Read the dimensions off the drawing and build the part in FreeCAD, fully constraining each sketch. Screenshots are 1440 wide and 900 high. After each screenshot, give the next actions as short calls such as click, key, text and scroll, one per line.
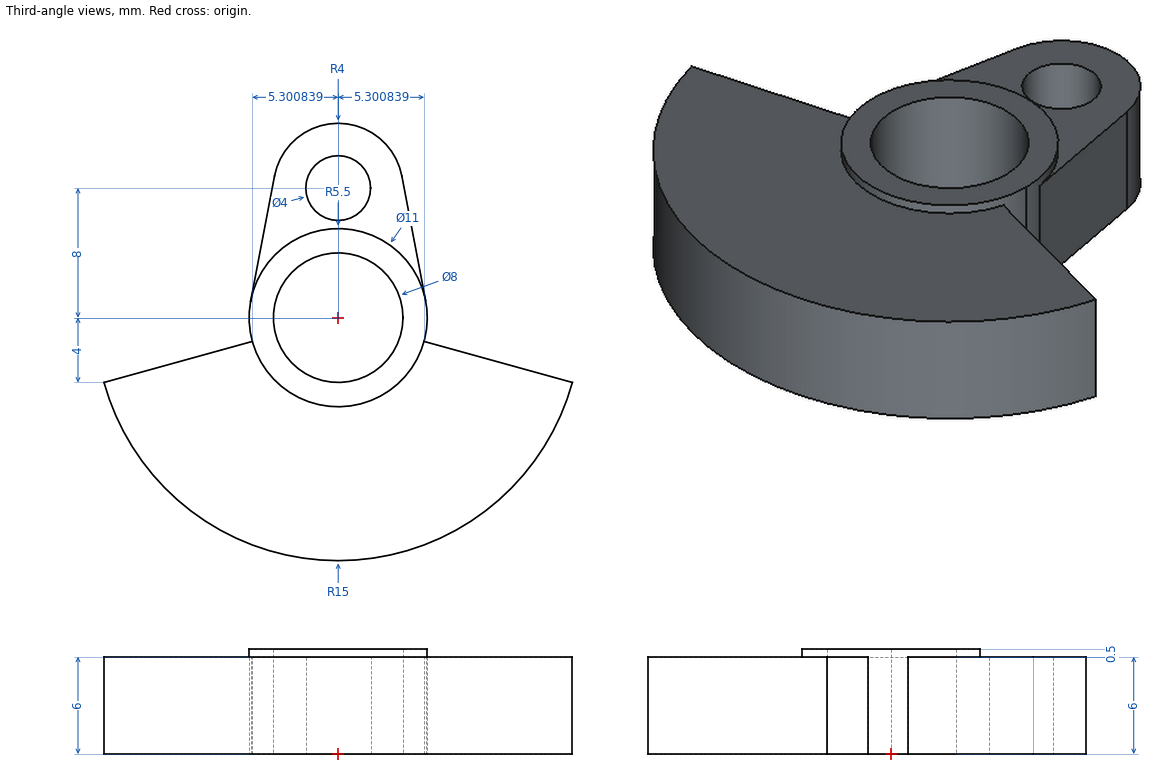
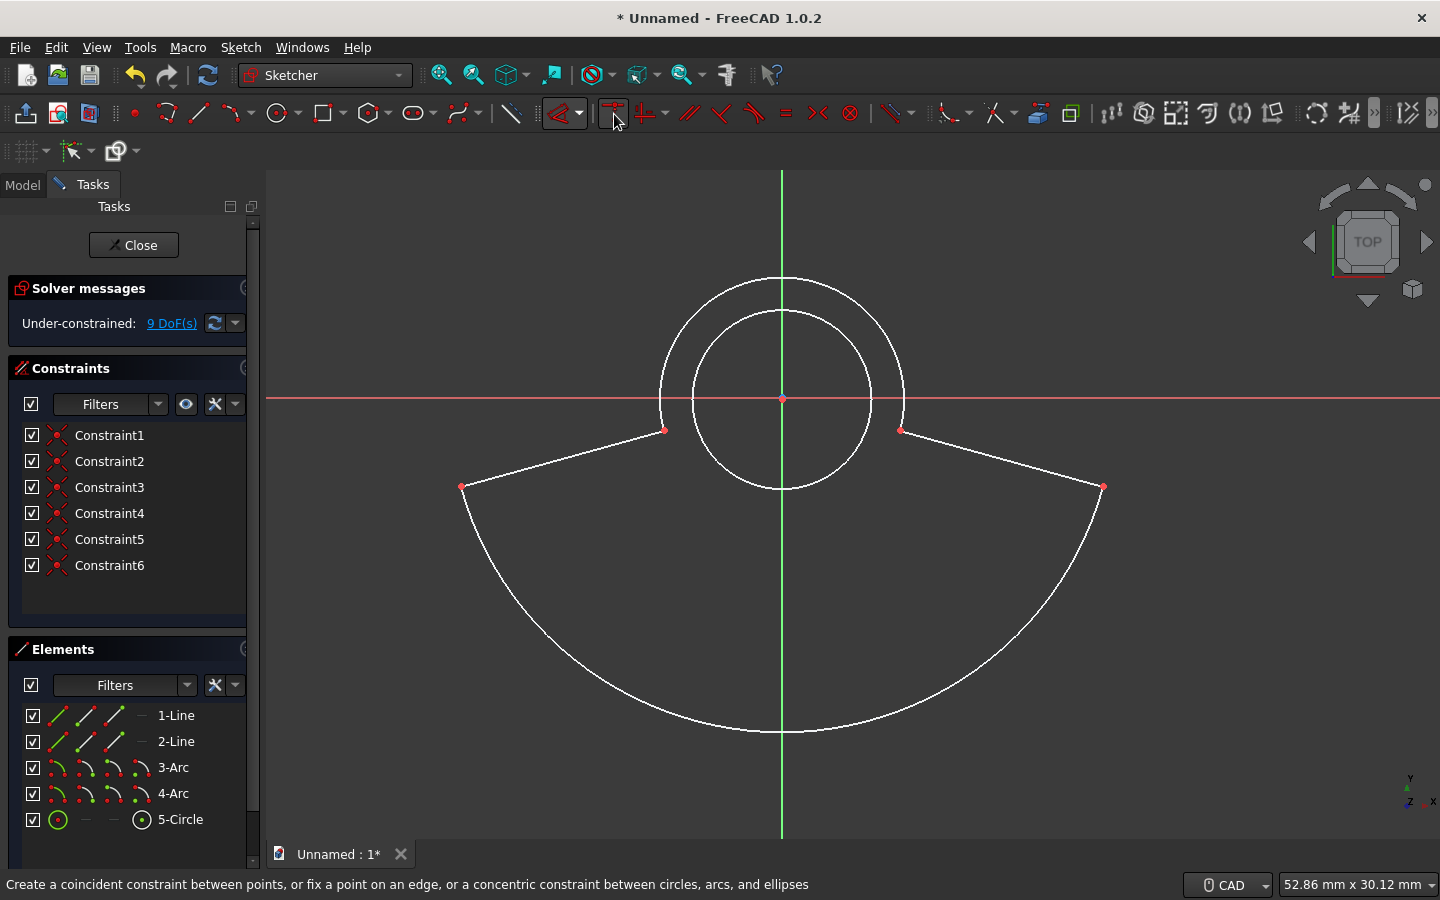
drag(772, 388, 792, 410)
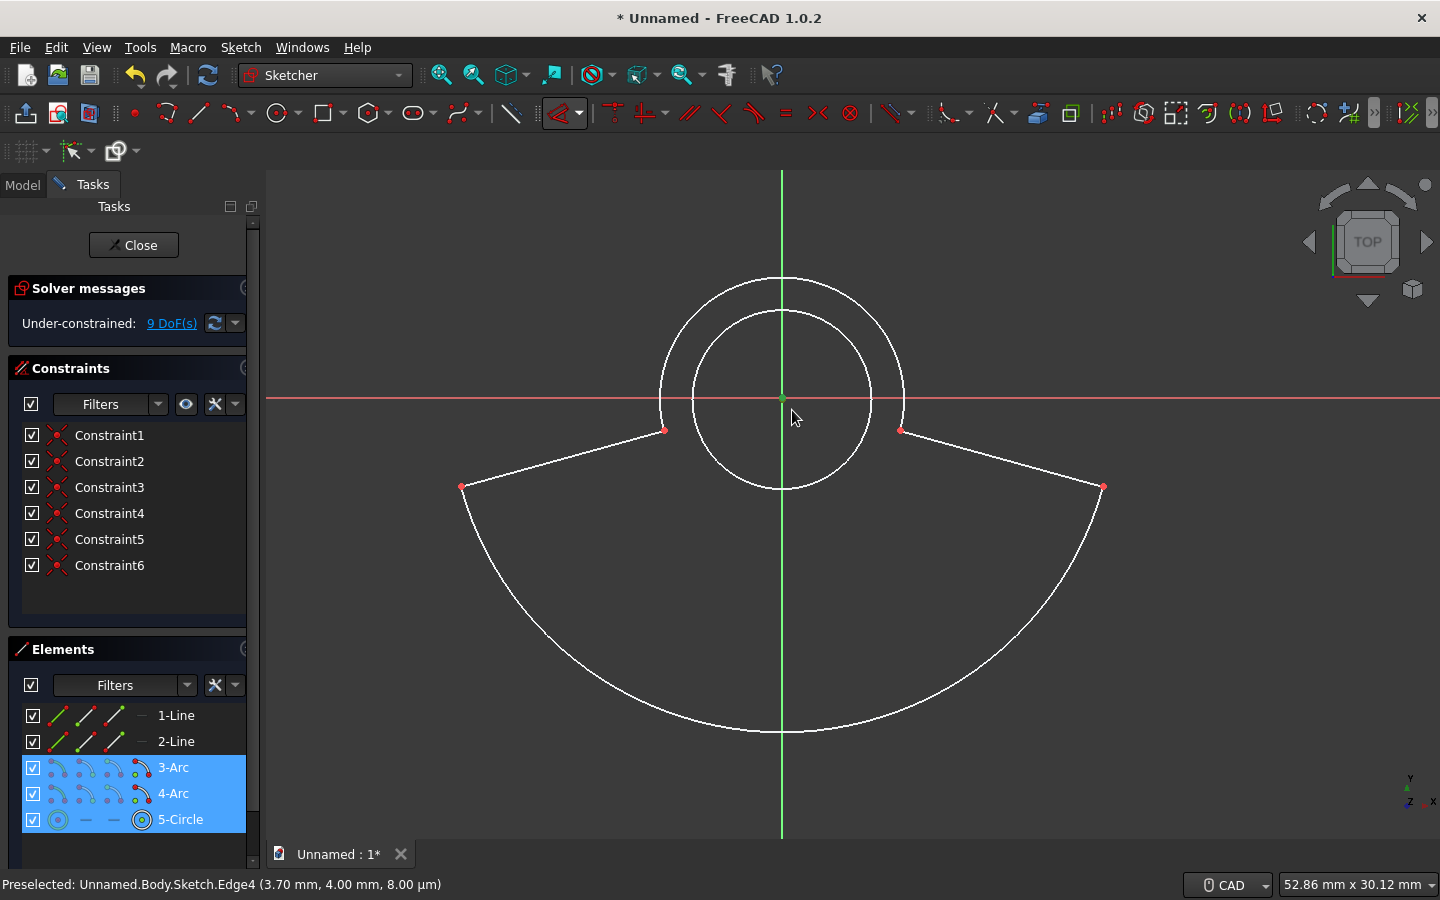
click(614, 114)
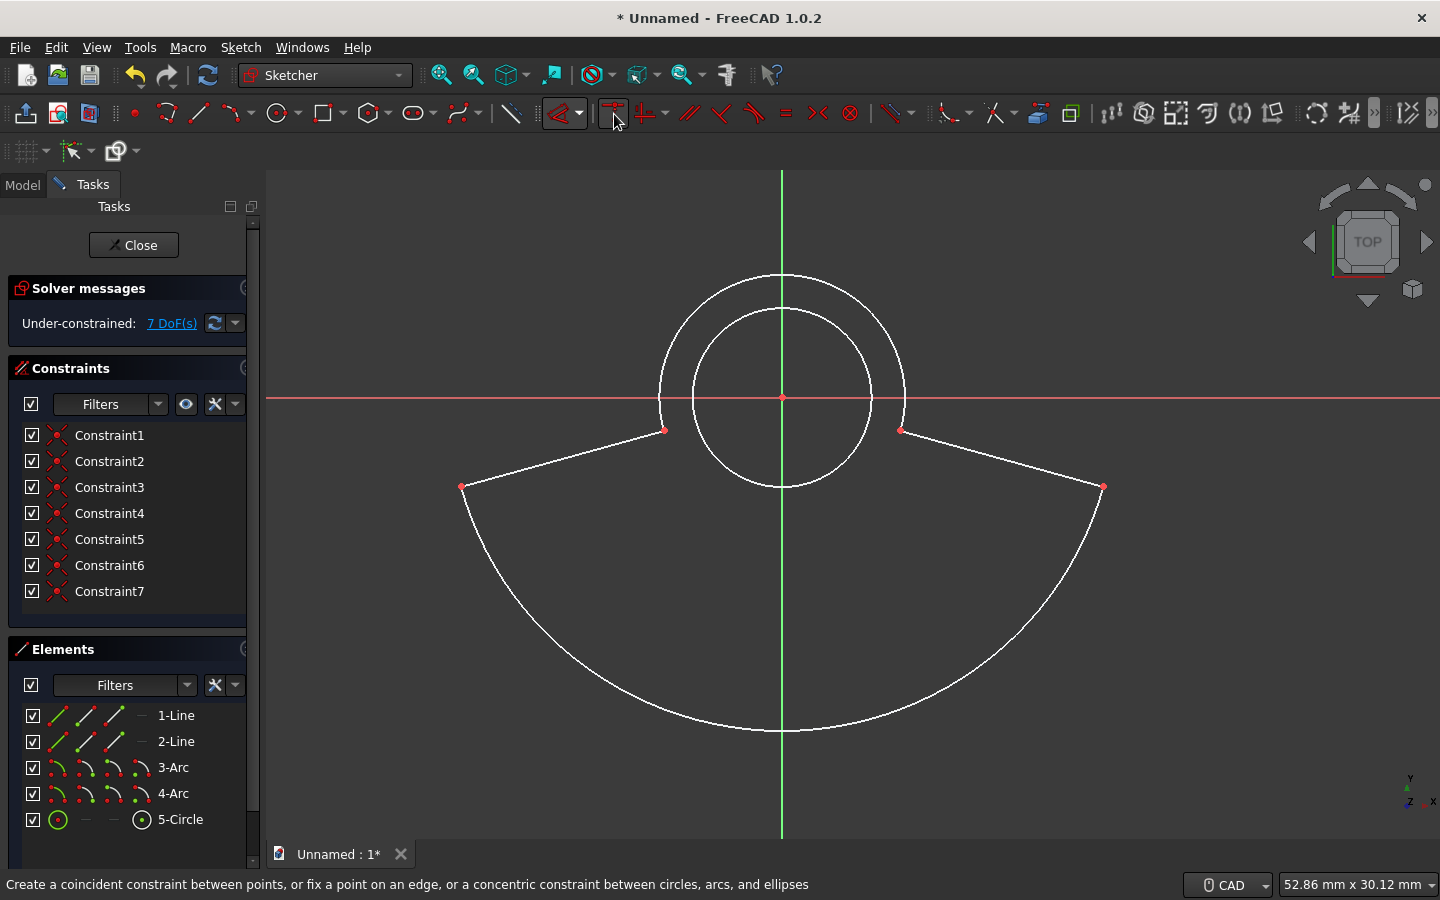
click(558, 114)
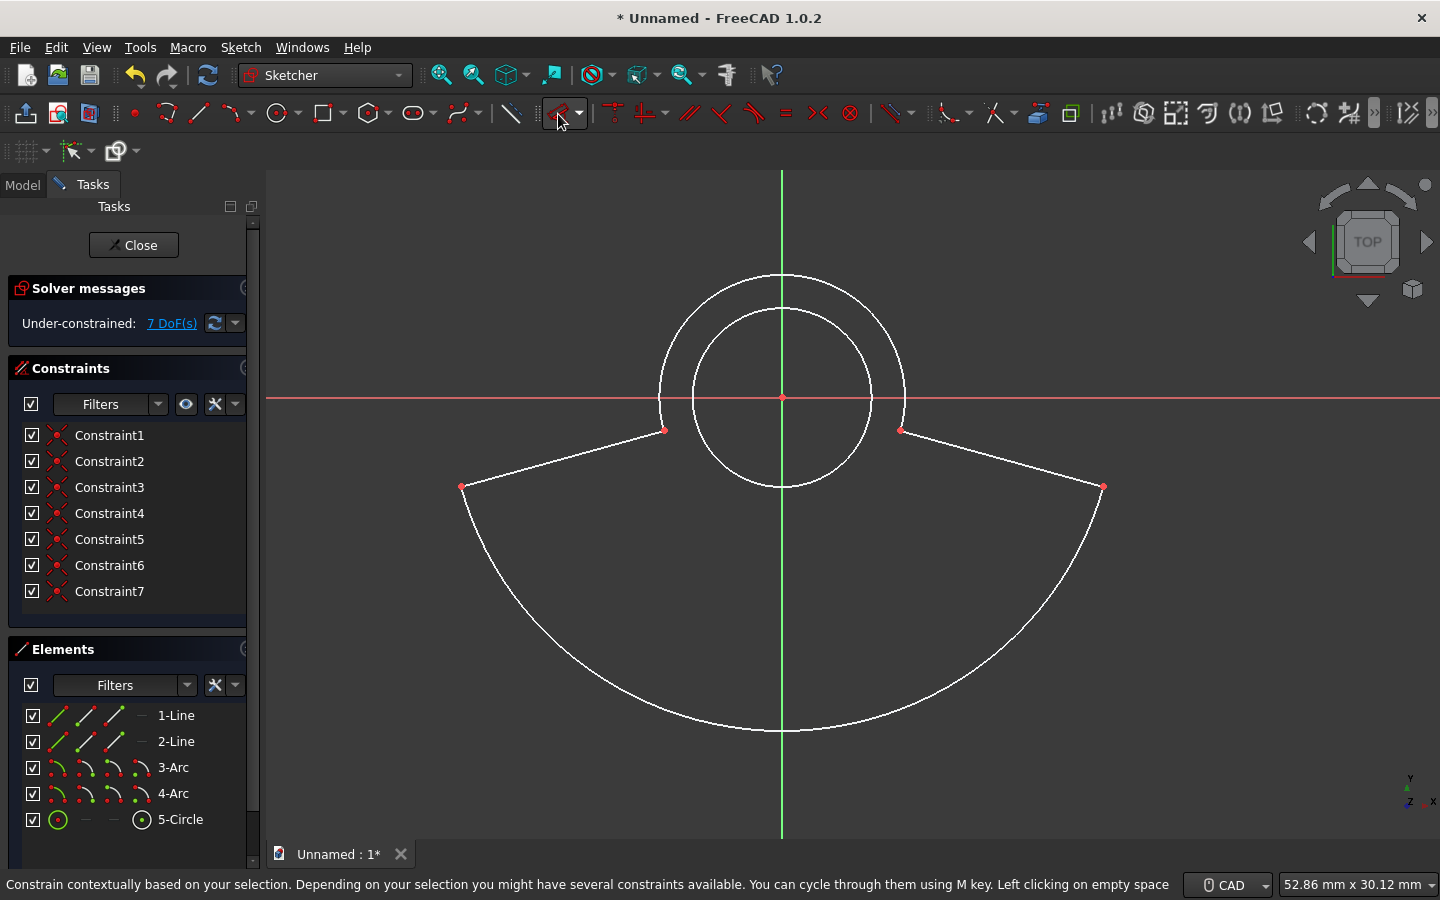
click(617, 687)
click(601, 715)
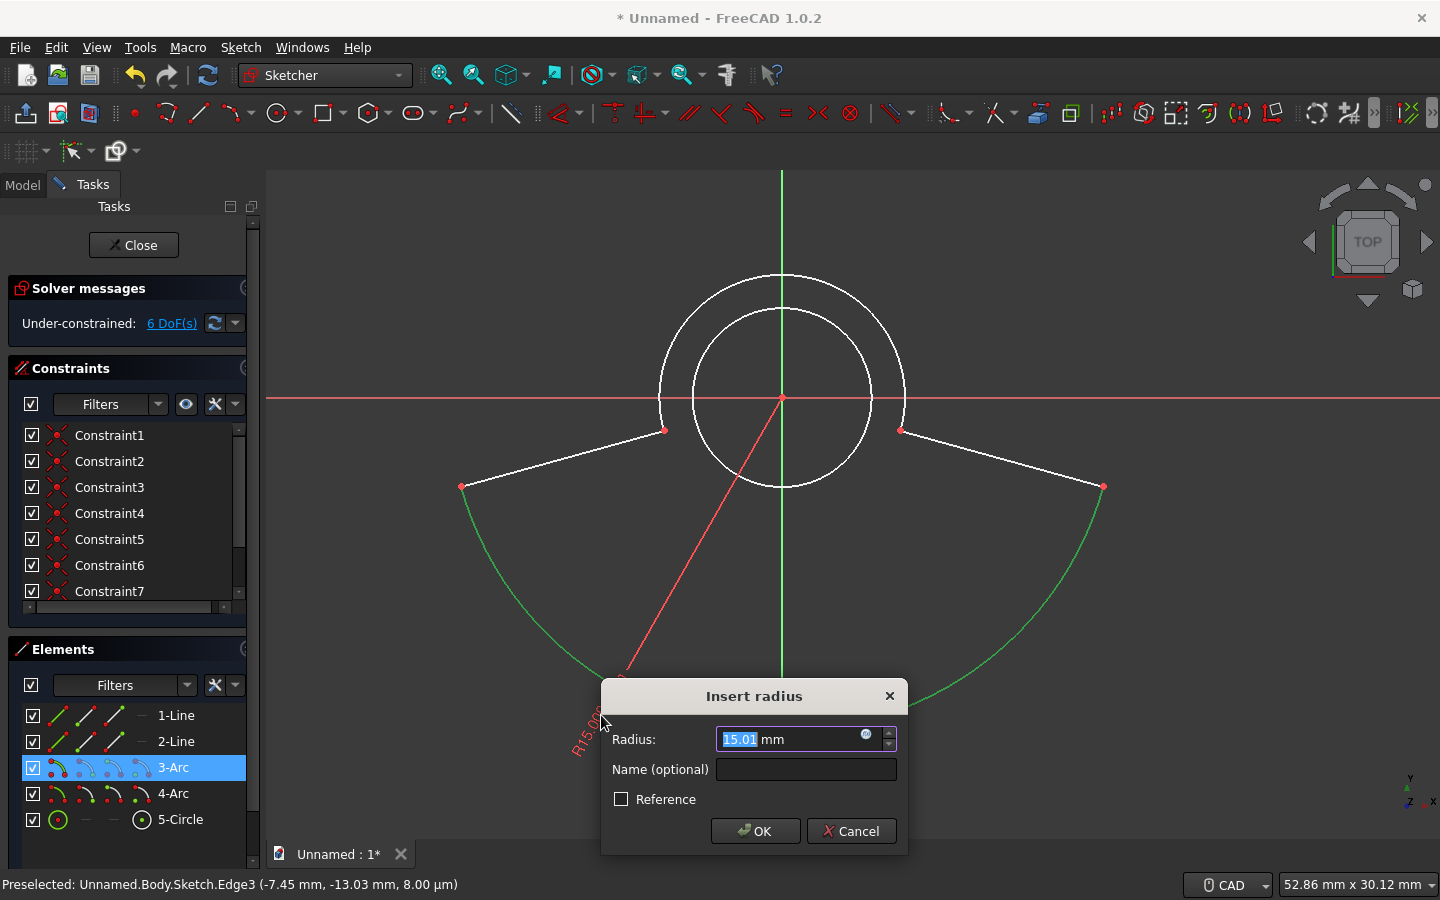
text(15)
key(Return)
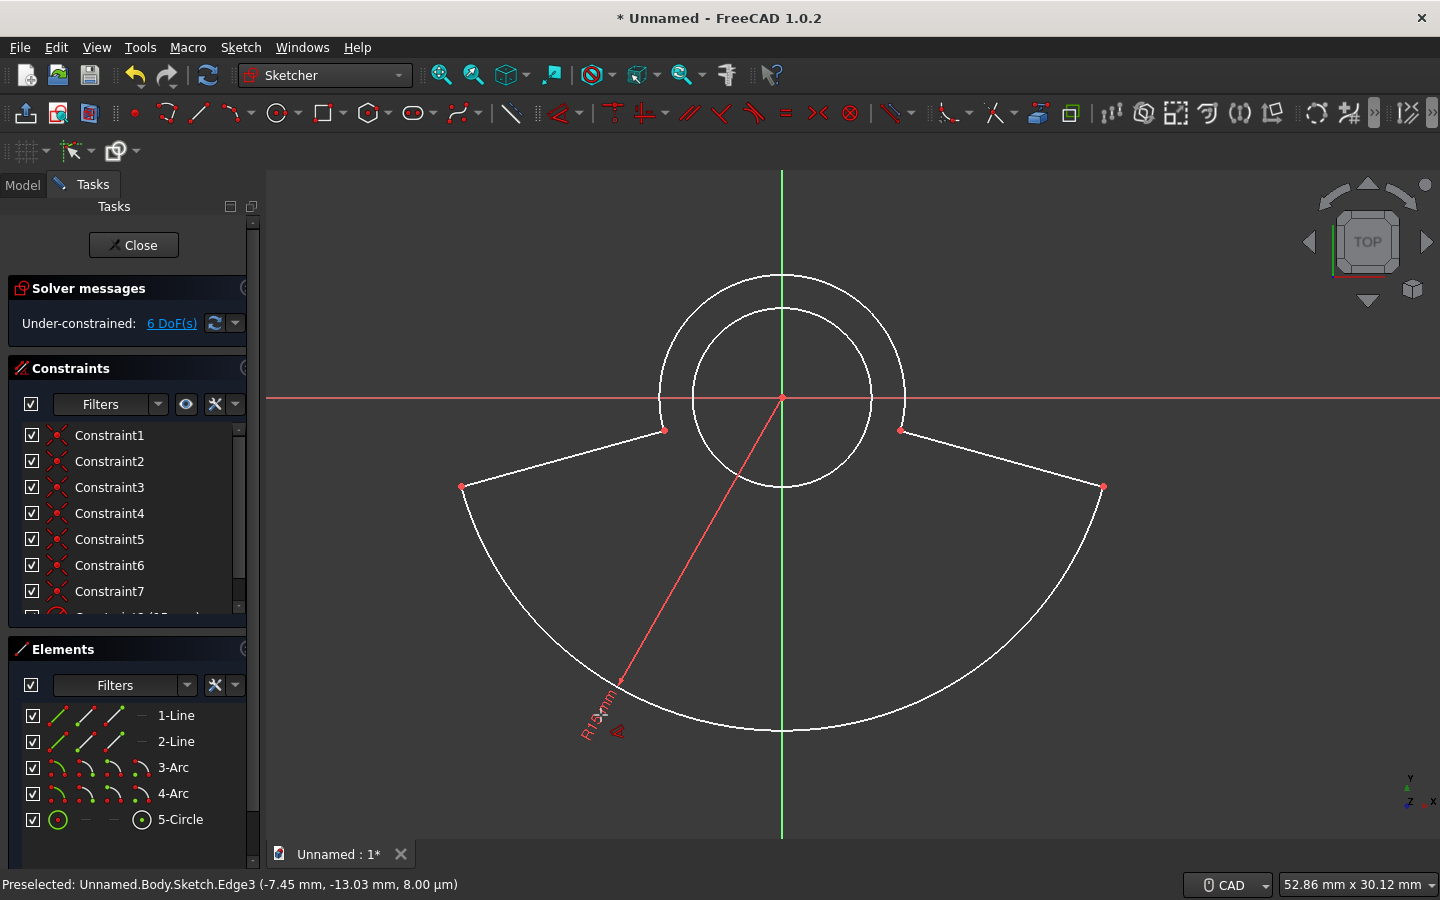
click(865, 307)
click(887, 283)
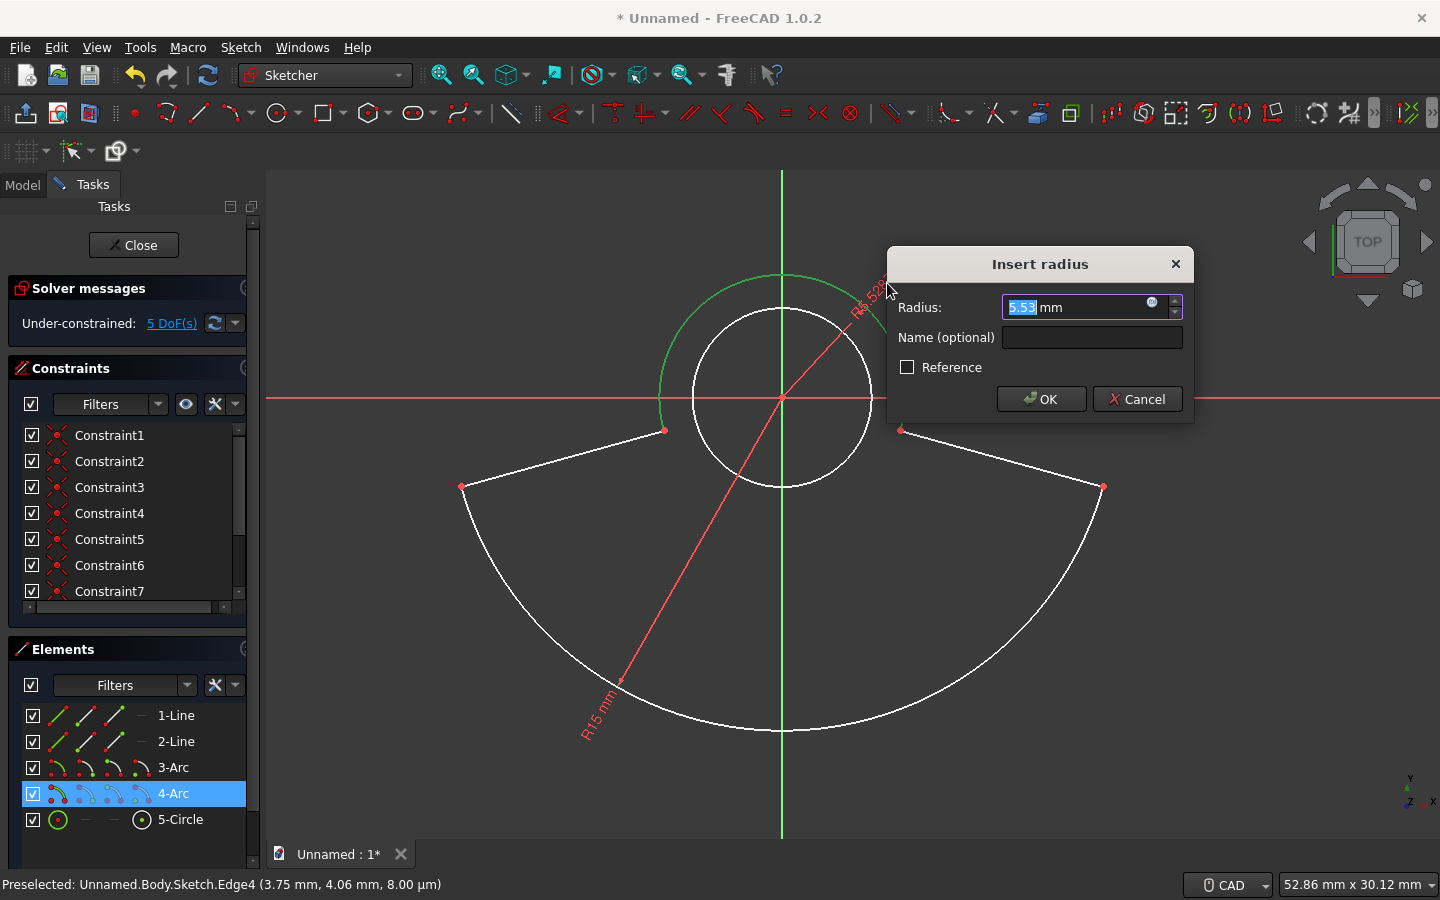
text(5.5)
key(Return)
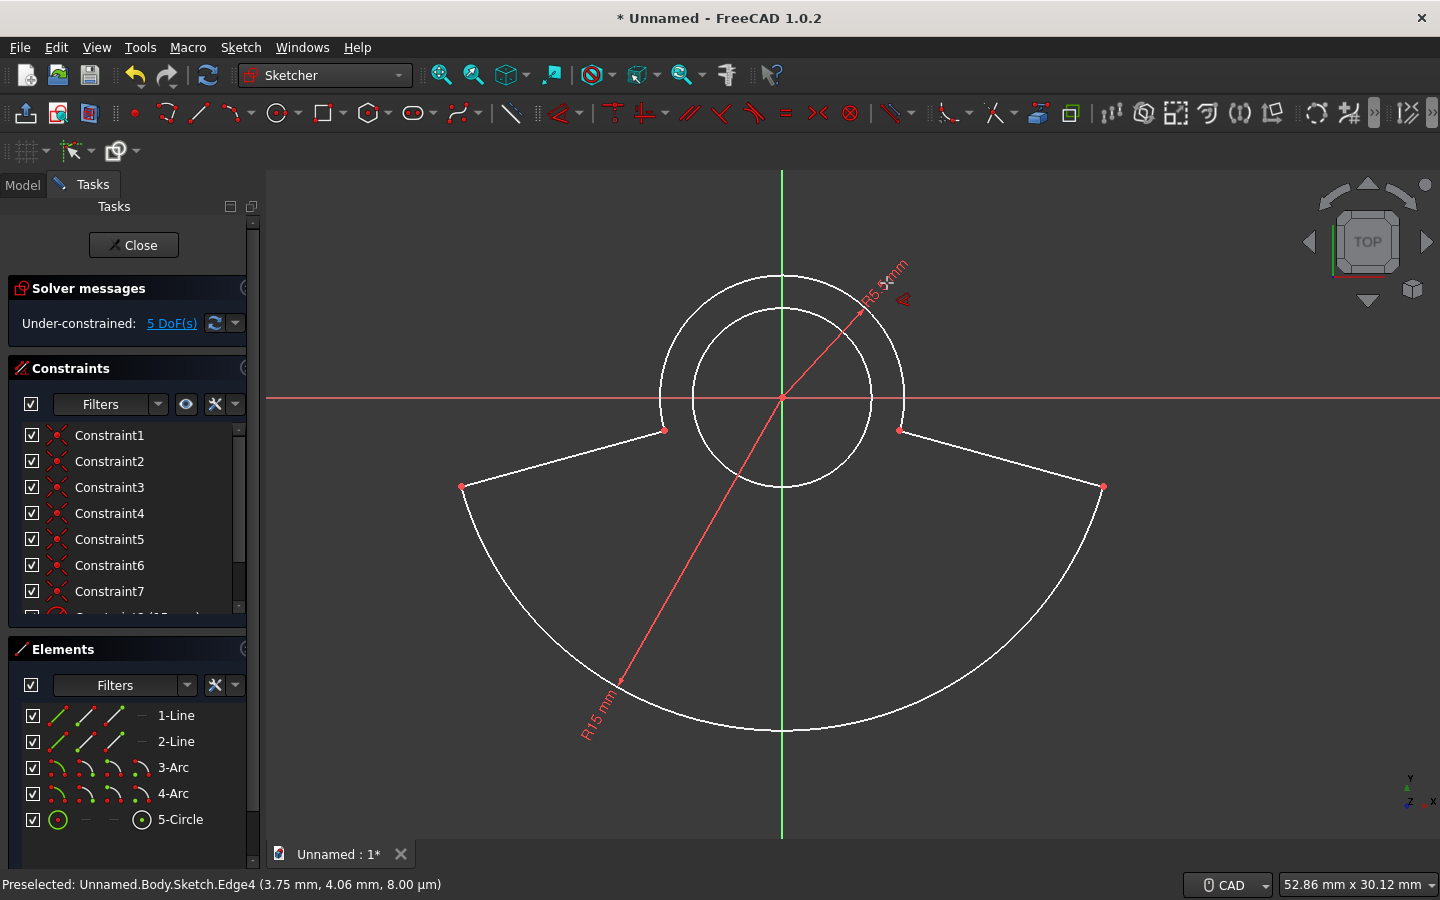
click(845, 334)
click(869, 483)